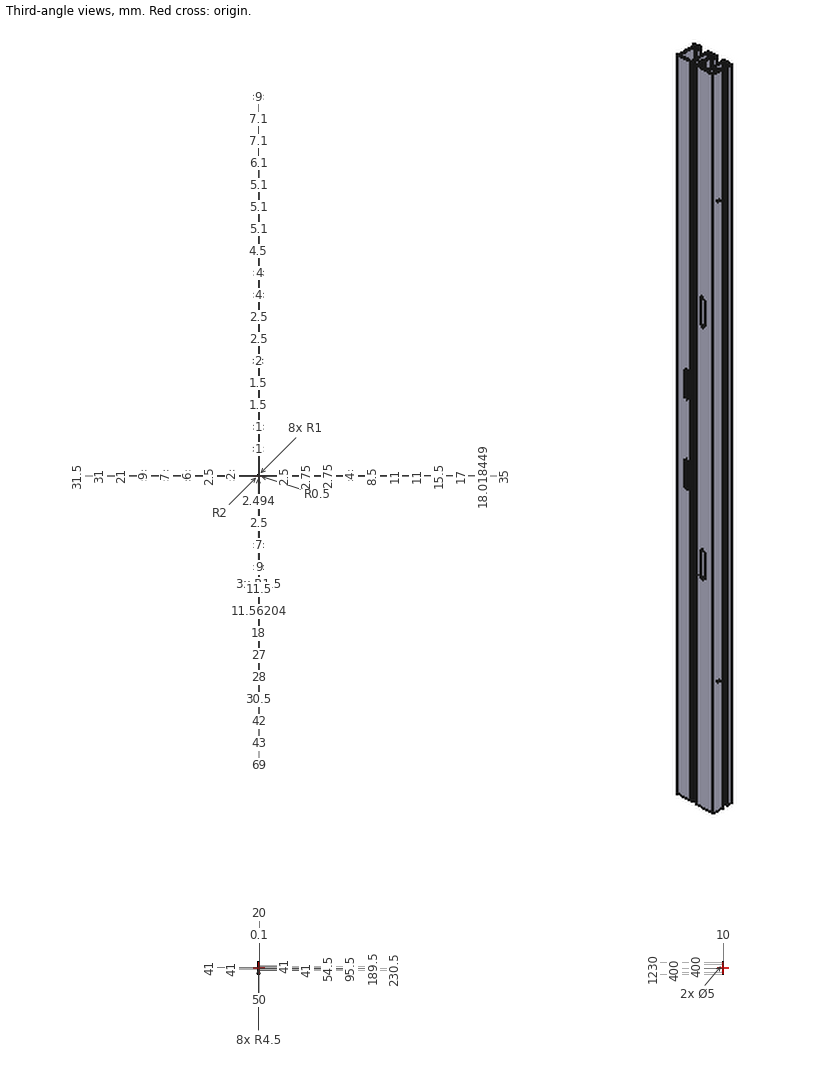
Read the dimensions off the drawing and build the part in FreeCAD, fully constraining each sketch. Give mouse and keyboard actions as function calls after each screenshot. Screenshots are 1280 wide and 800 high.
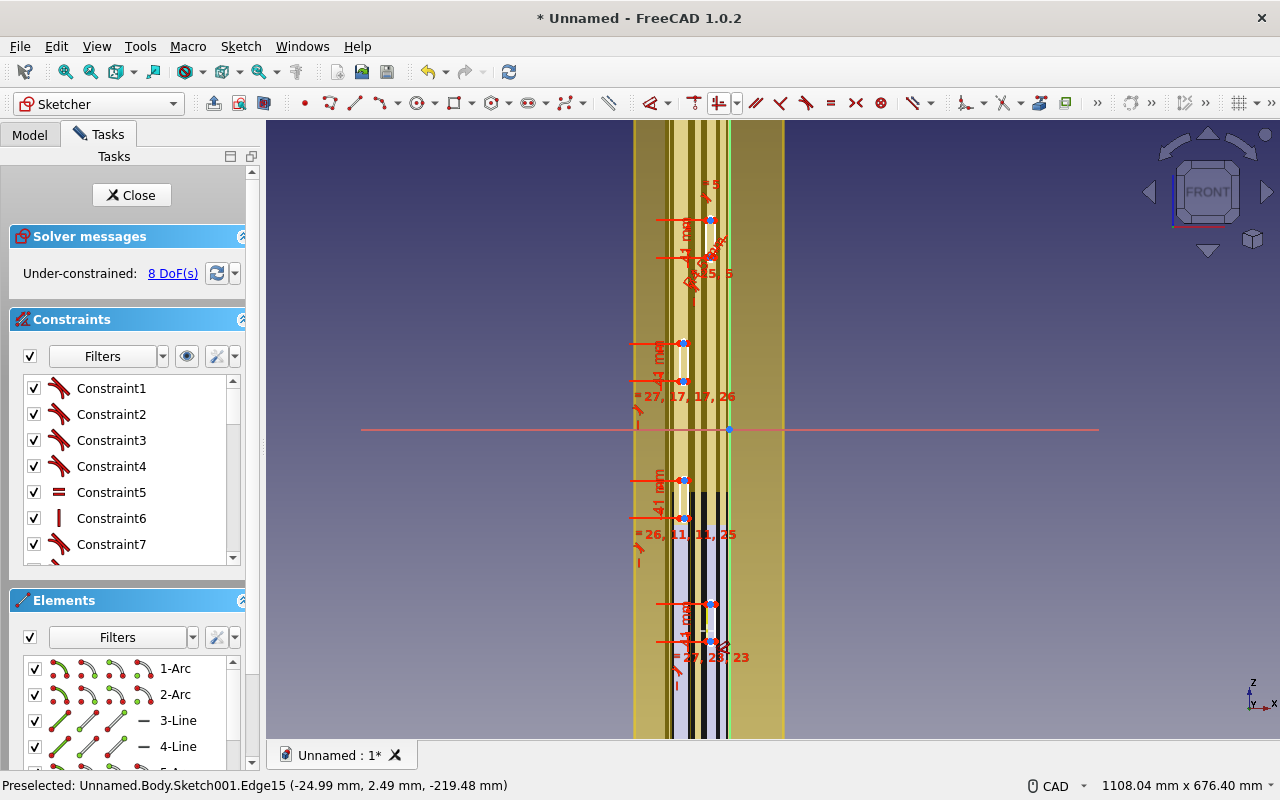
scroll(711, 258, up, 6)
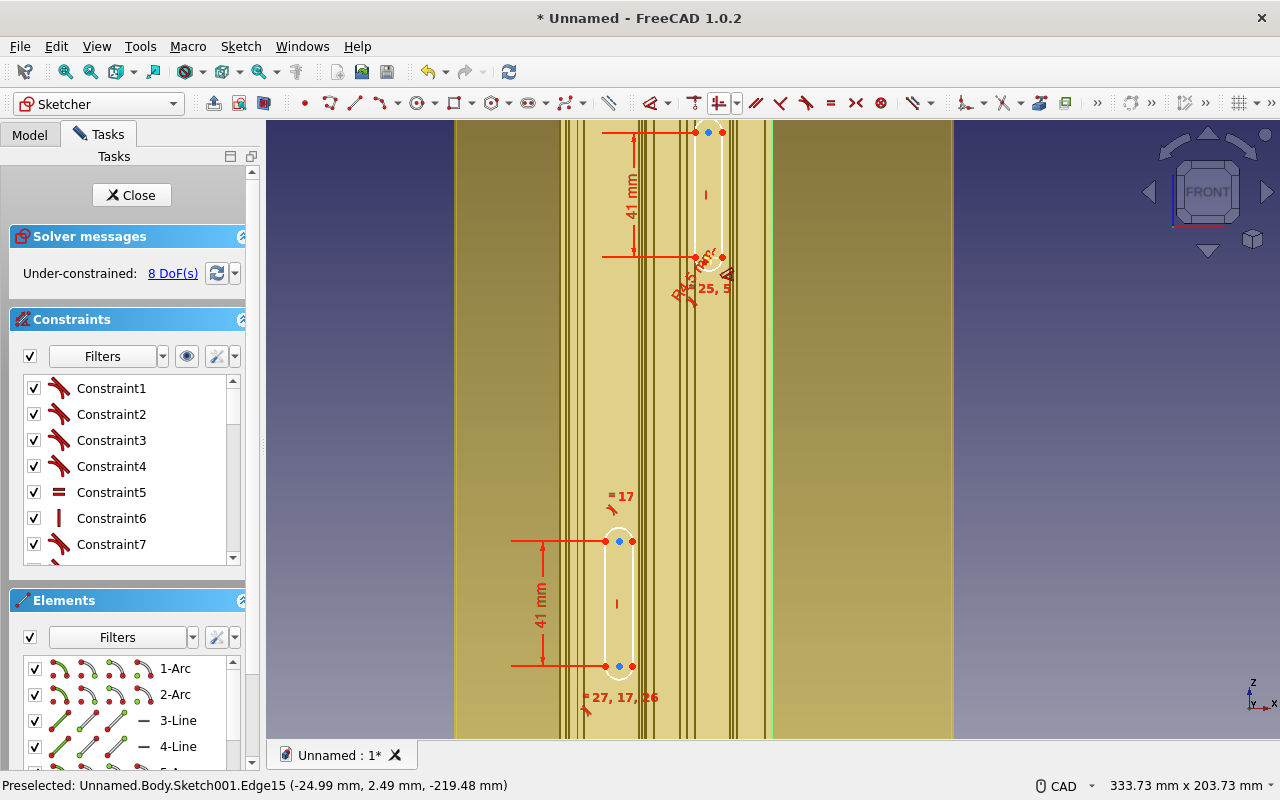
click(709, 257)
click(740, 223)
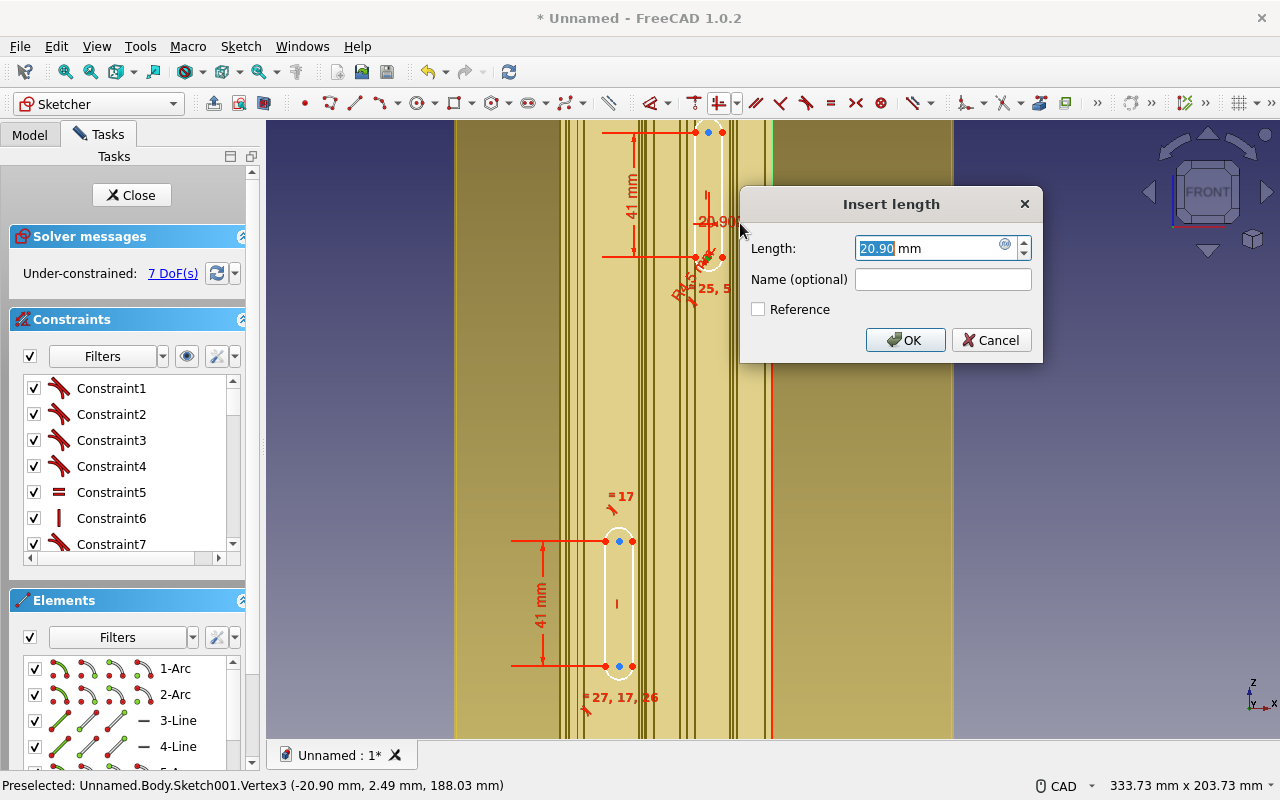
text(20)
key(Return)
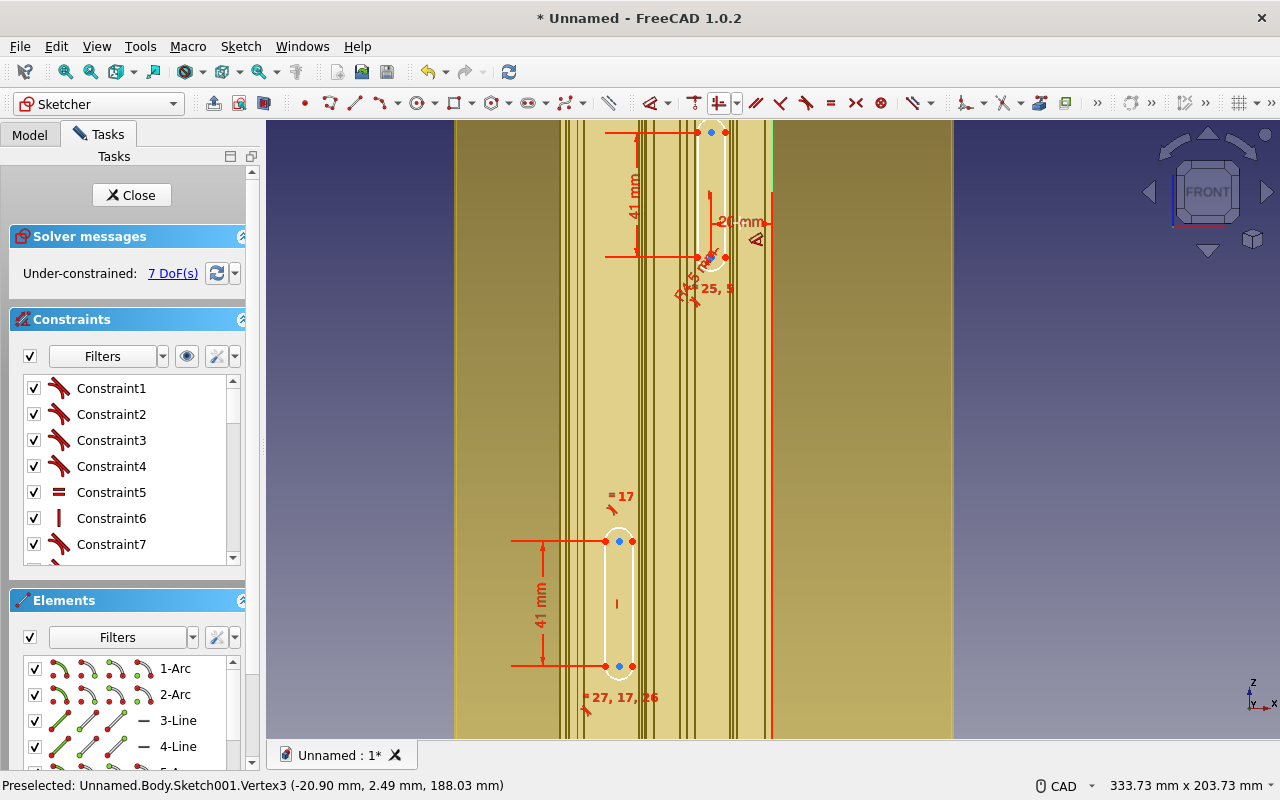
scroll(711, 258, down, 6)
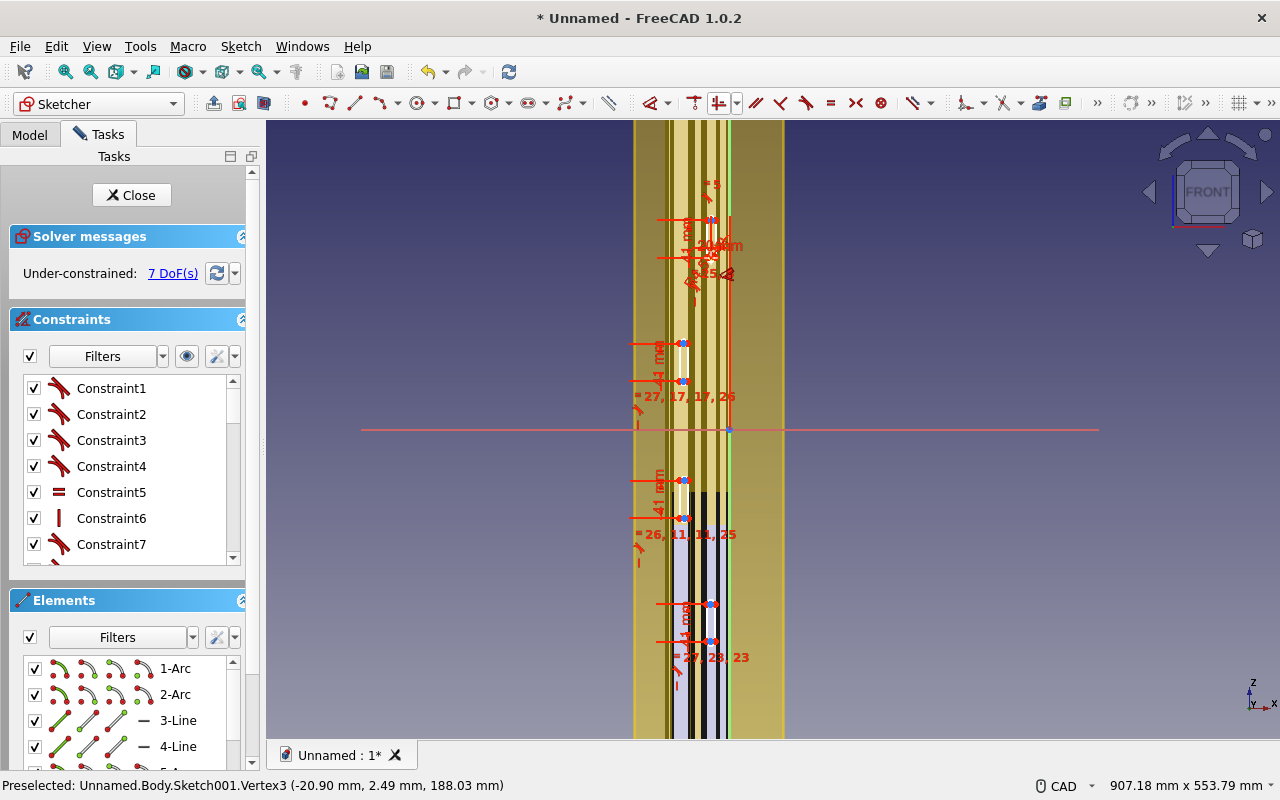
scroll(684, 518, up, 6)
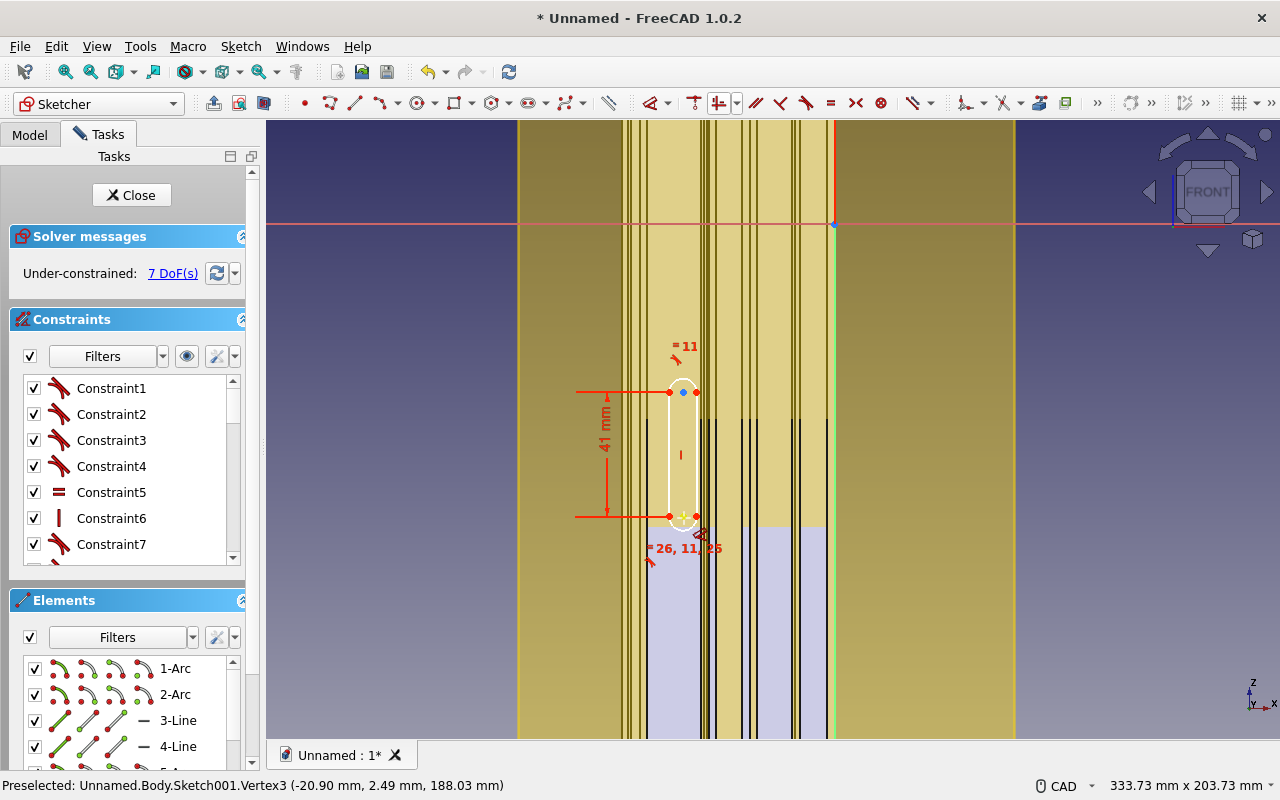
click(683, 517)
click(759, 551)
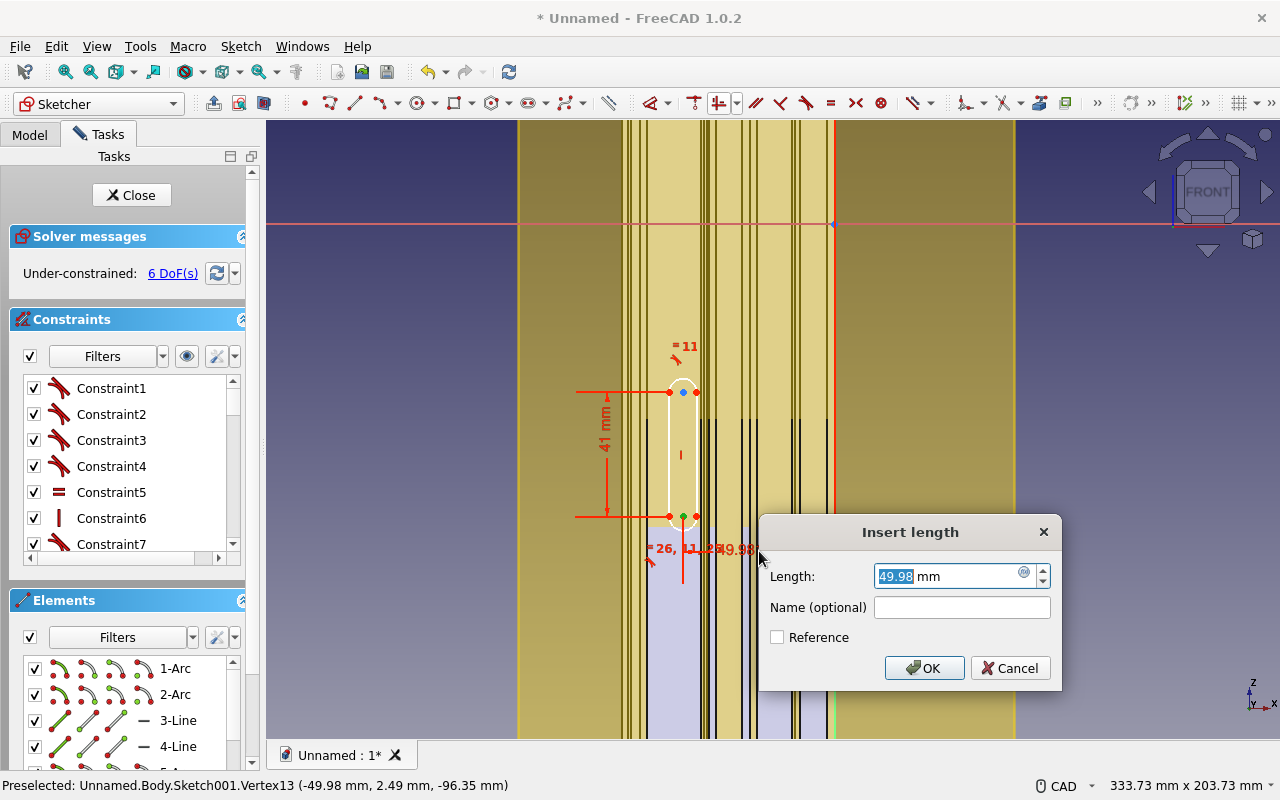
text(50)
key(Return)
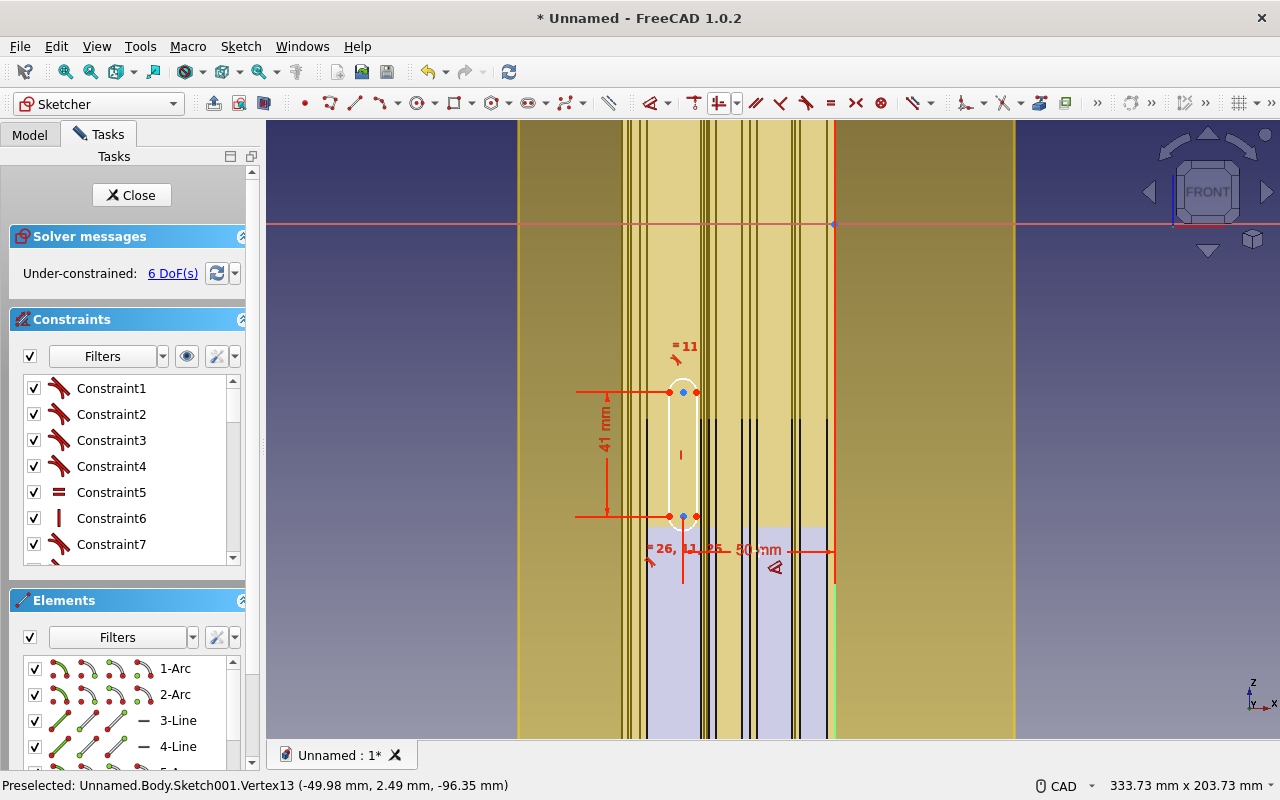
scroll(684, 518, down, 6)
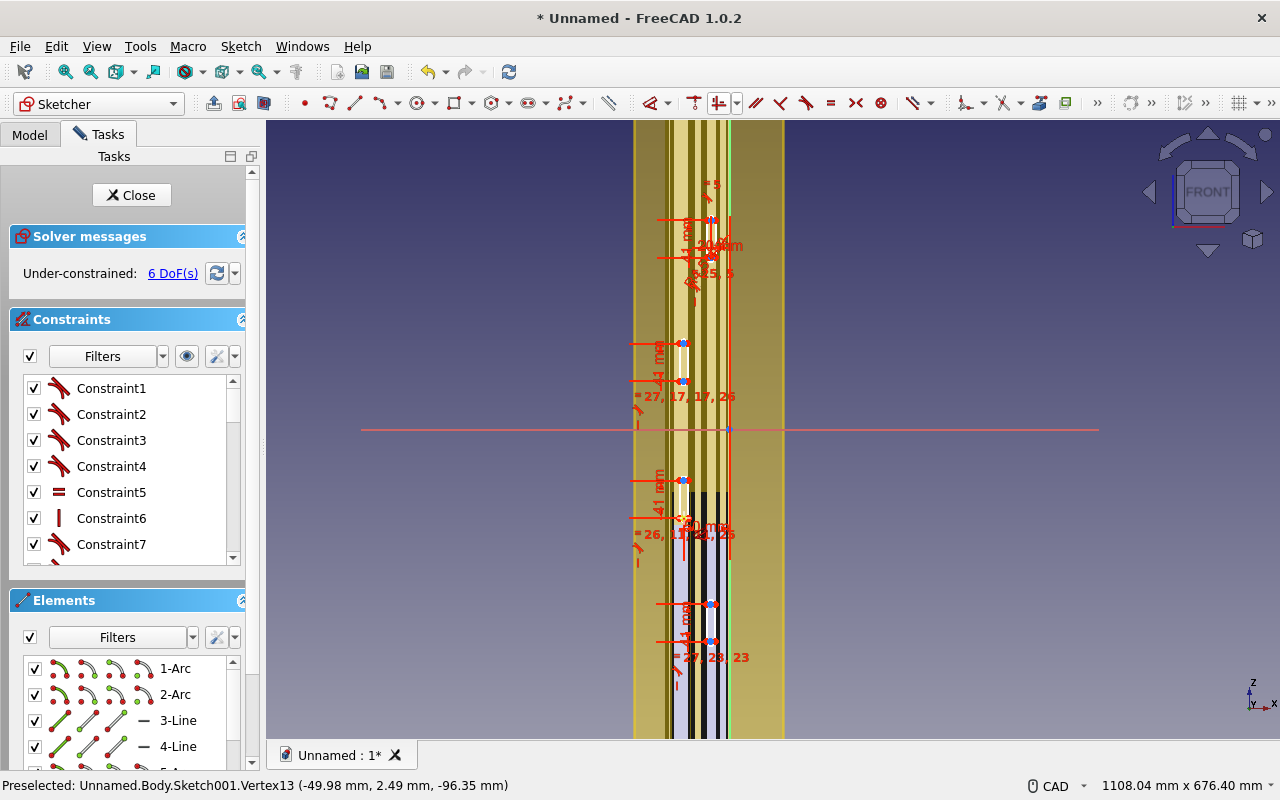
scroll(684, 381, up, 6)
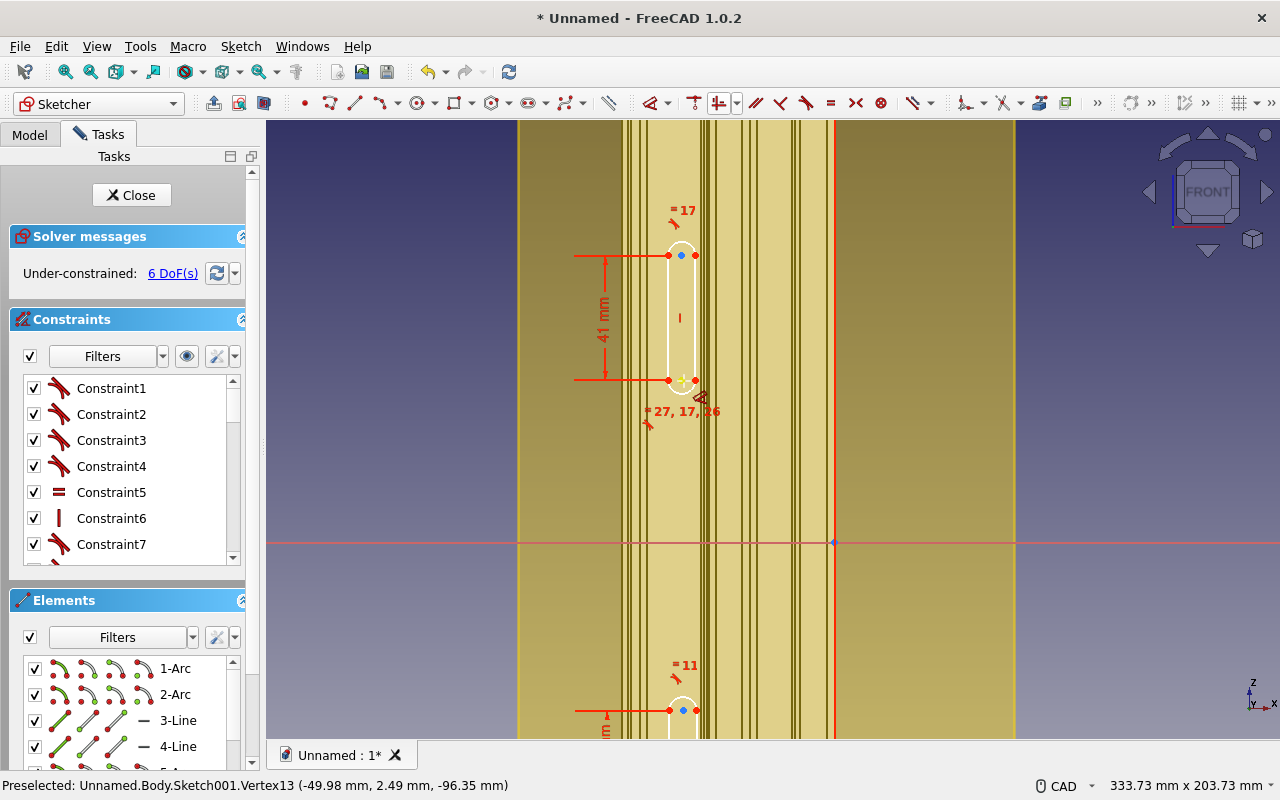
click(682, 380)
click(758, 346)